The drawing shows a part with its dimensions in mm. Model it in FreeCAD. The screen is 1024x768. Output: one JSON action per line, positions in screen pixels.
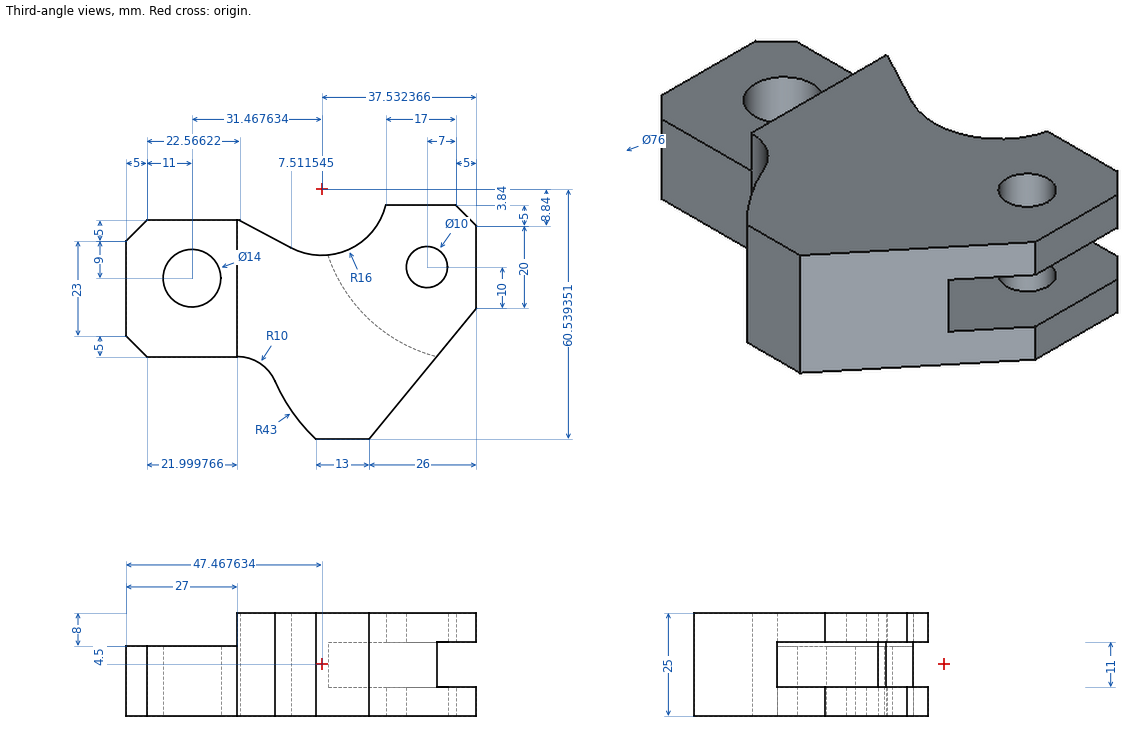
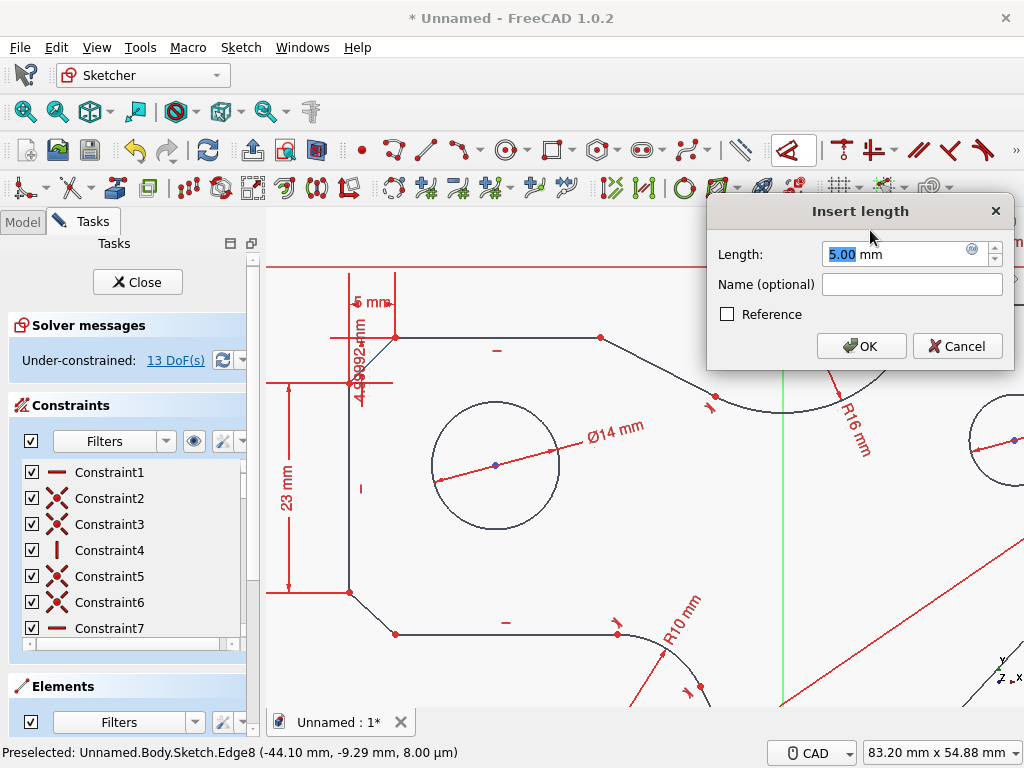
{"action": "type", "text": "5"}
{"action": "key", "text": "Return"}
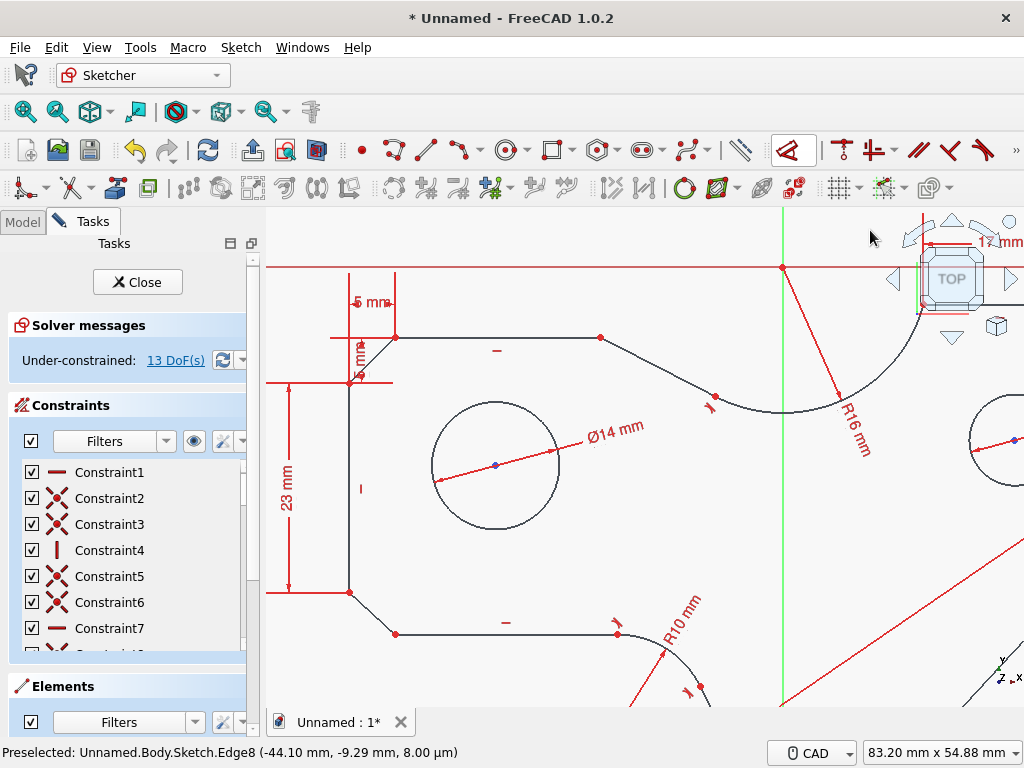
{"action": "left_click", "coordinate": [363, 605]}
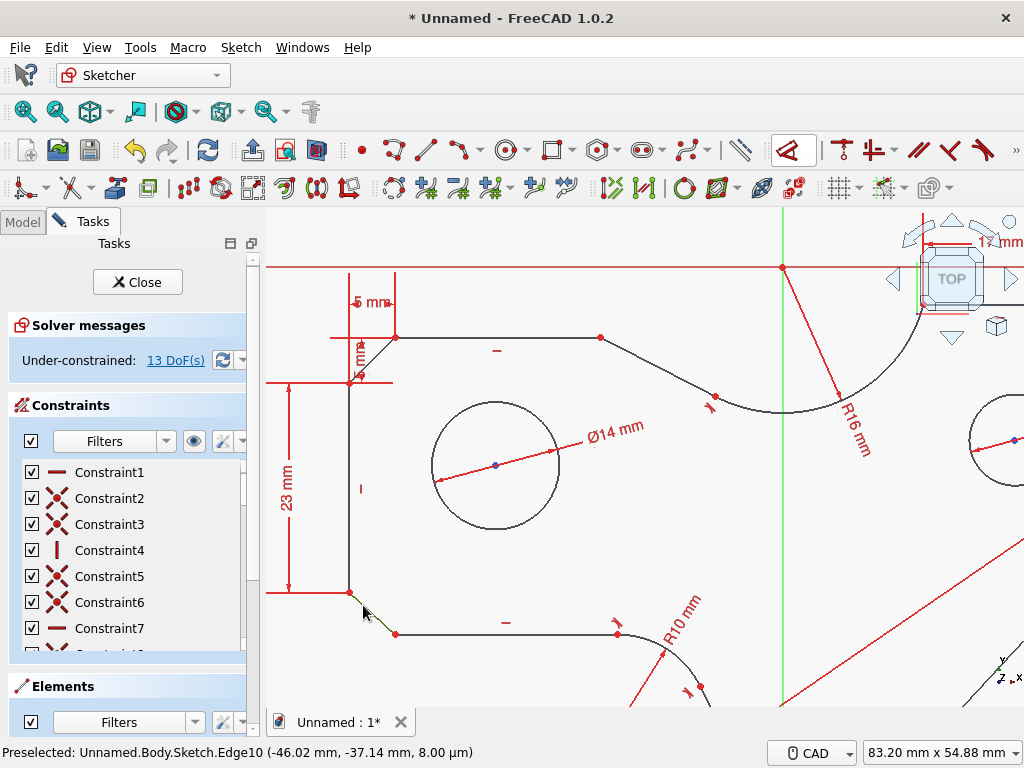
{"action": "key", "text": "l"}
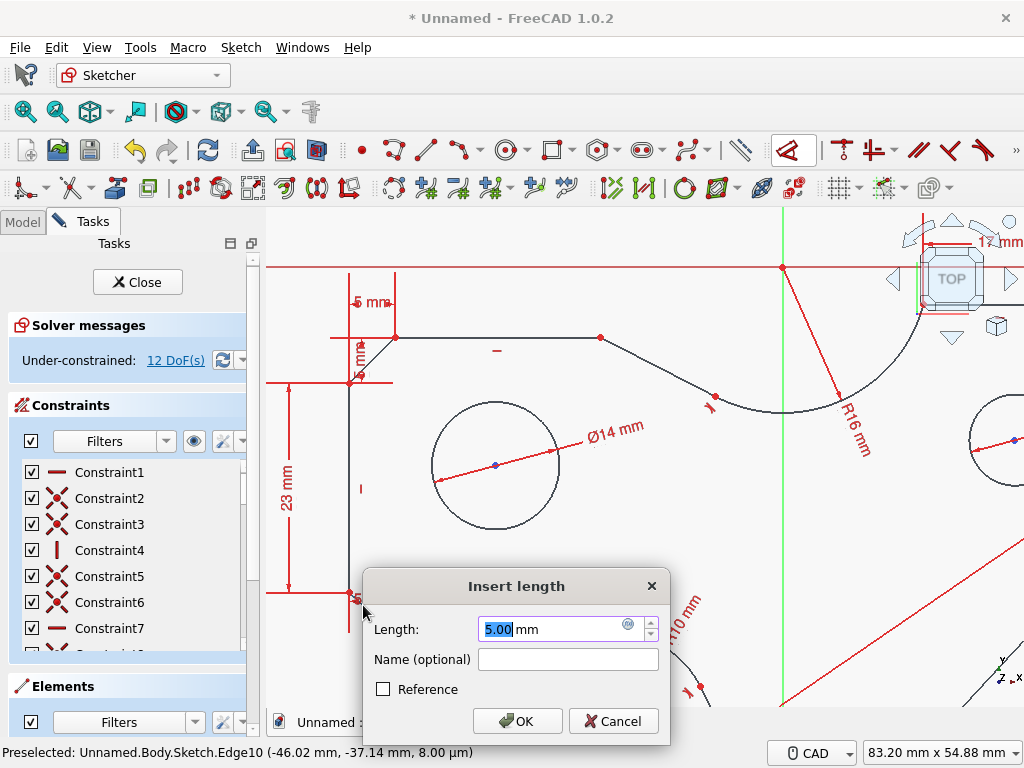
{"action": "type", "text": "5"}
{"action": "key", "text": "Return"}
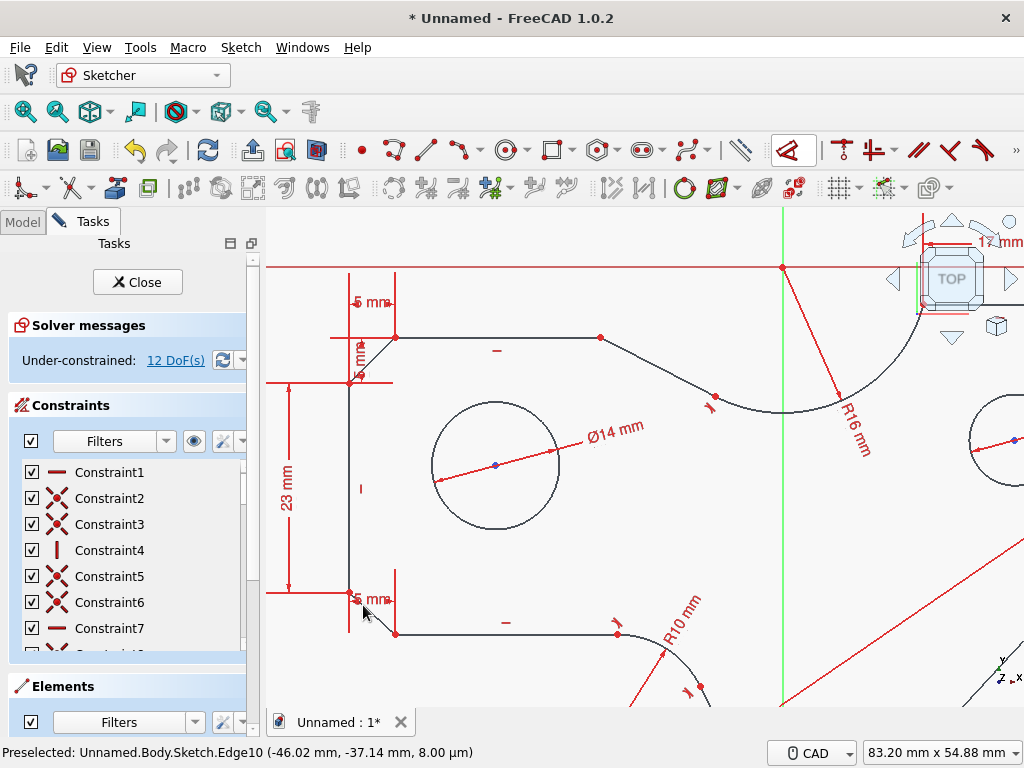
{"action": "left_click", "coordinate": [381, 622]}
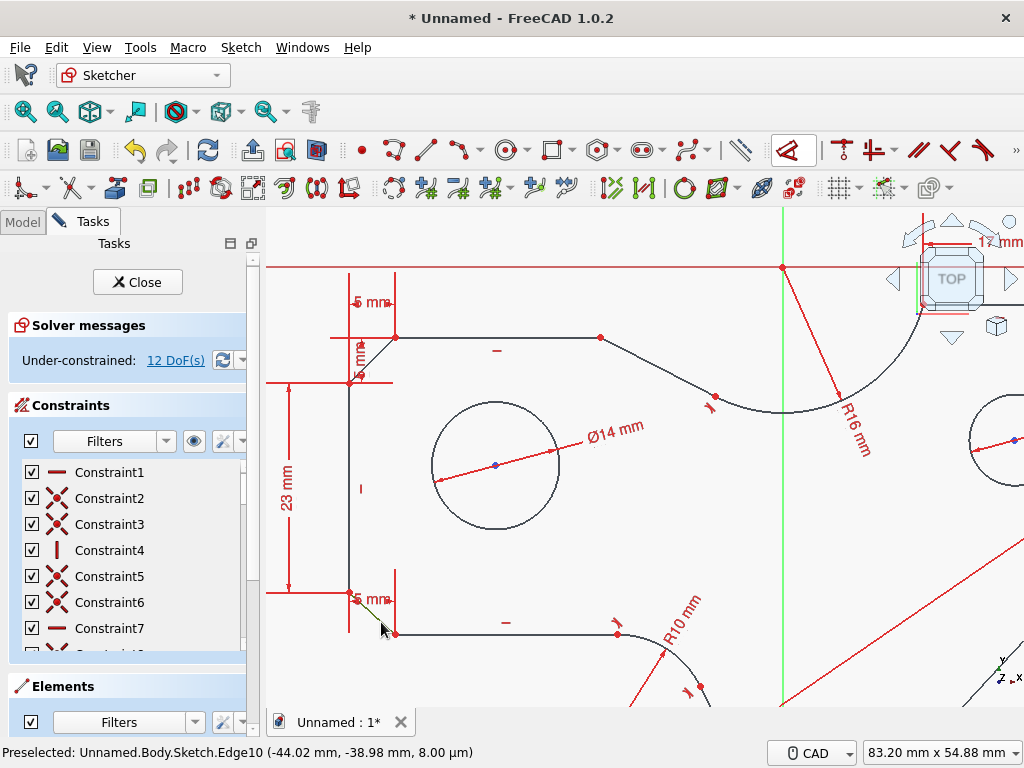
{"action": "left_click", "coordinate": [810, 150]}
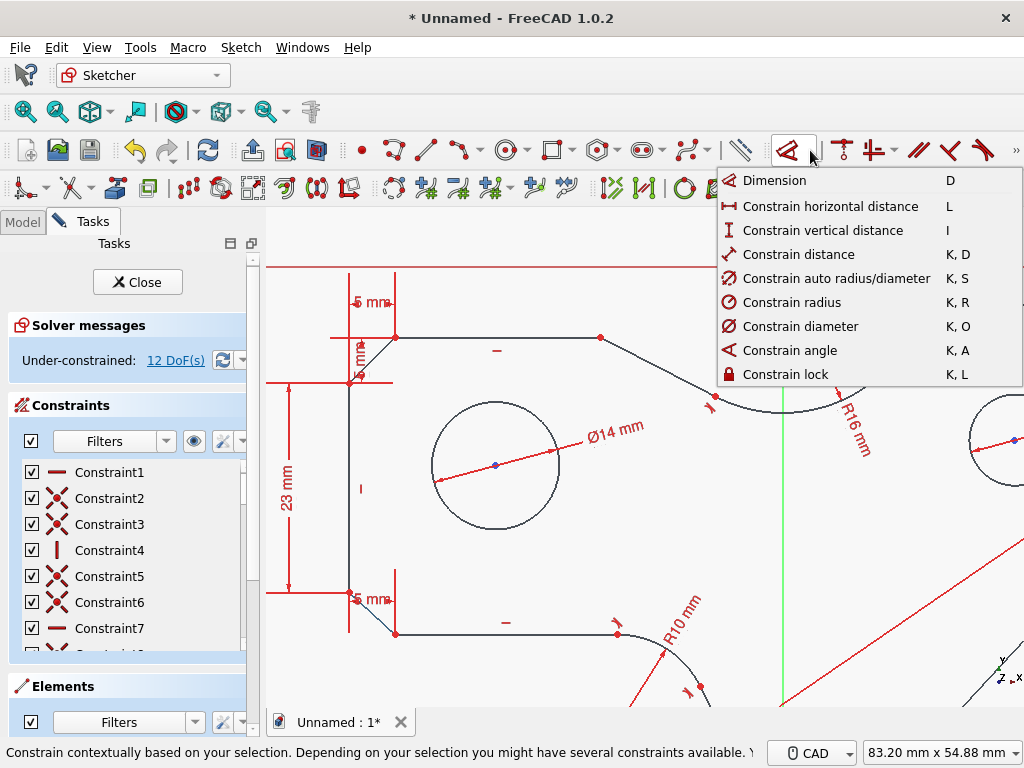
{"action": "left_click", "coordinate": [870, 230]}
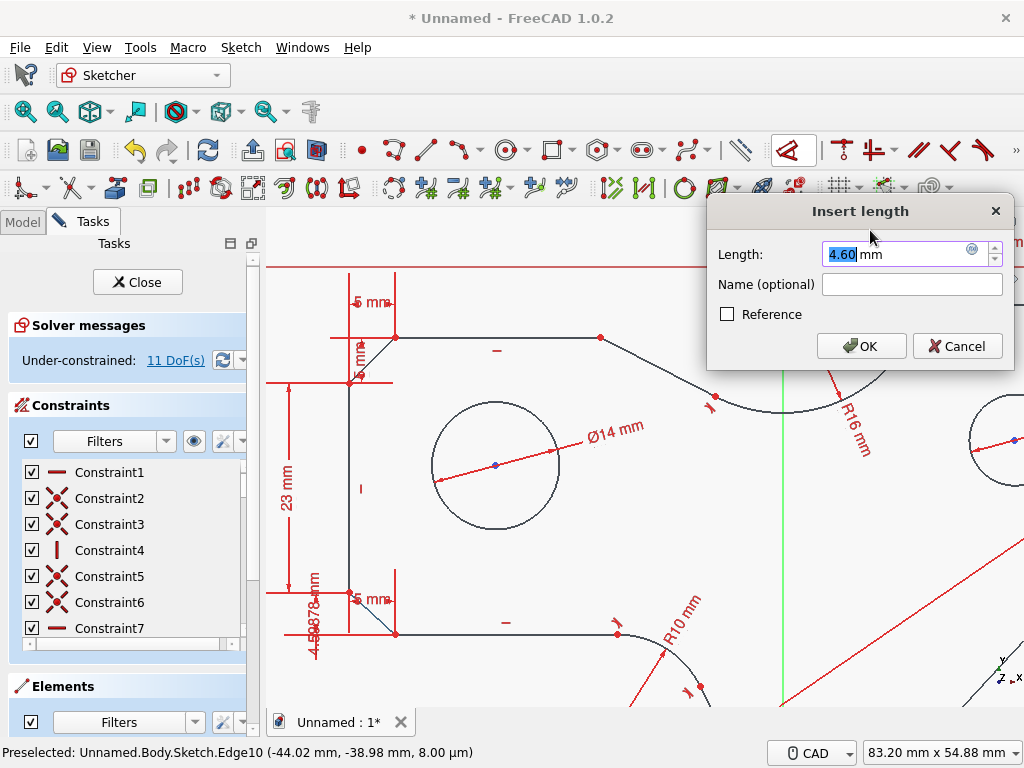
{"action": "type", "text": "5"}
{"action": "key", "text": "Return"}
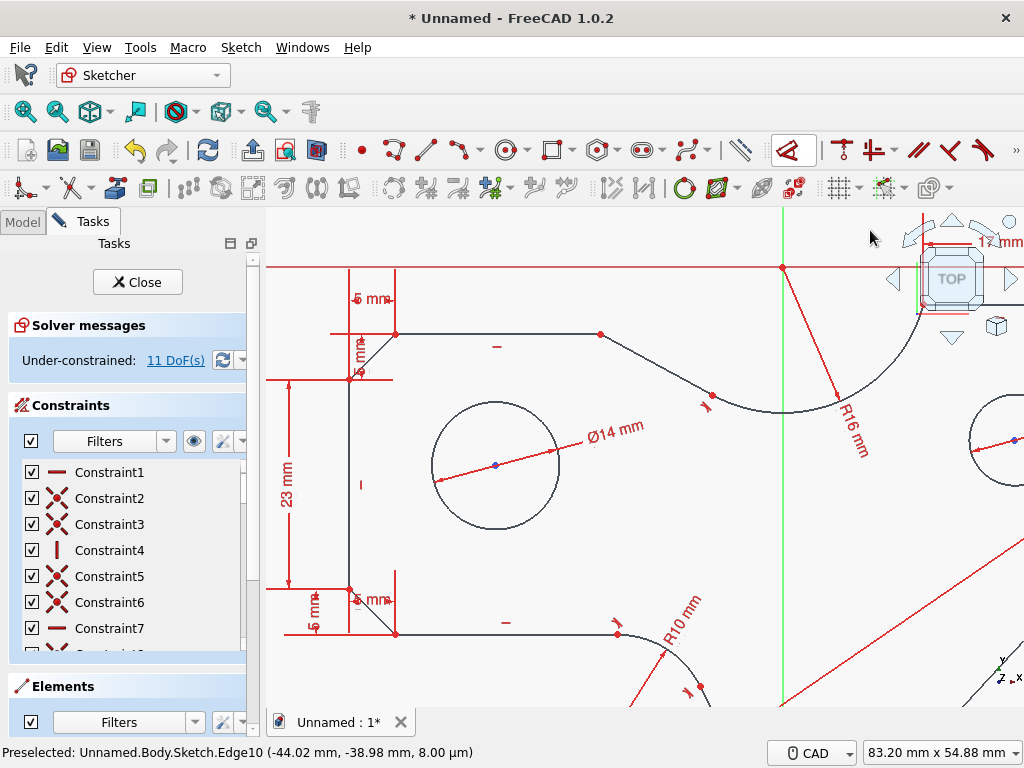
{"action": "left_click", "coordinate": [349, 380]}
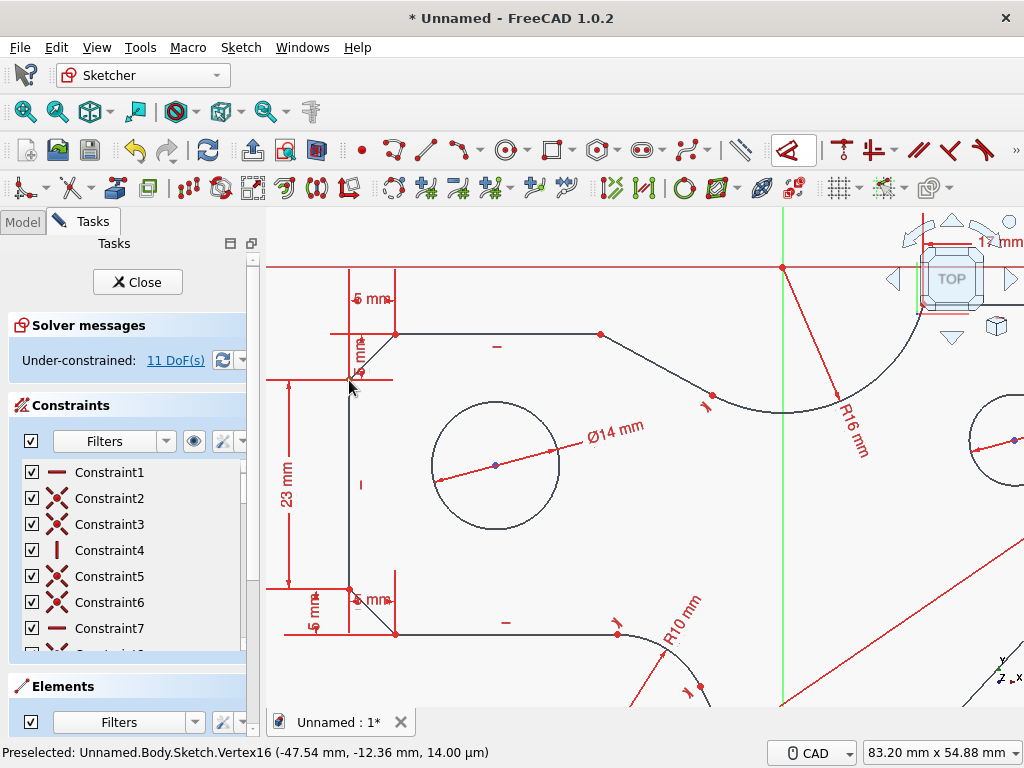
{"action": "left_click", "coordinate": [496, 466]}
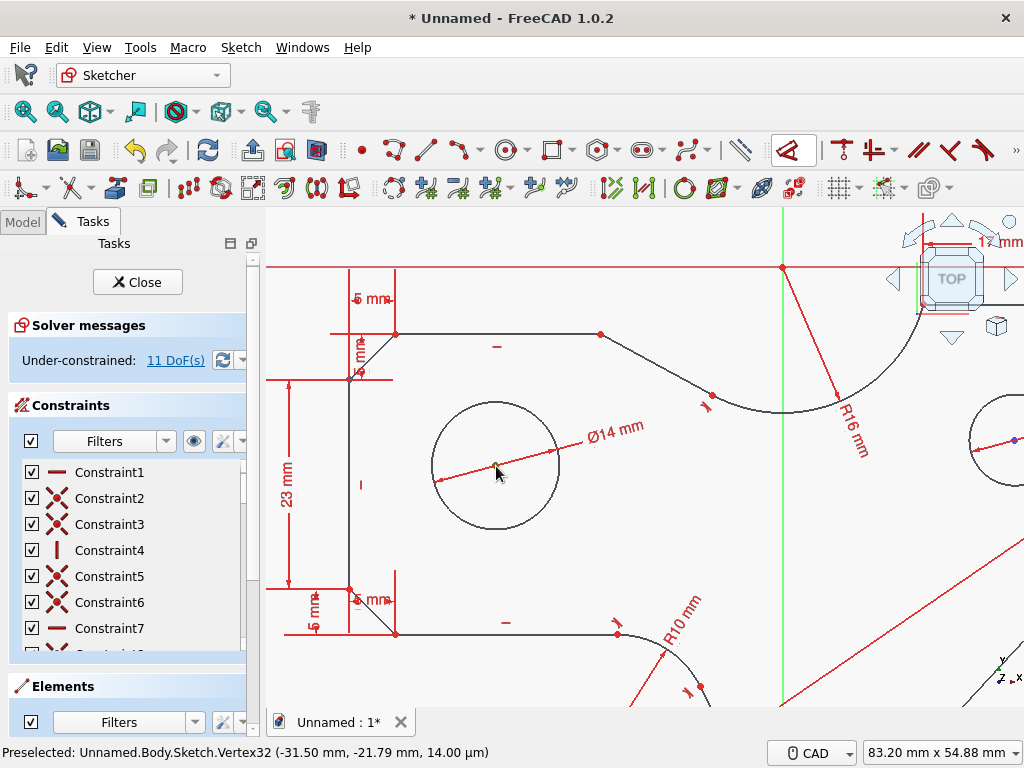
{"action": "key", "text": "i"}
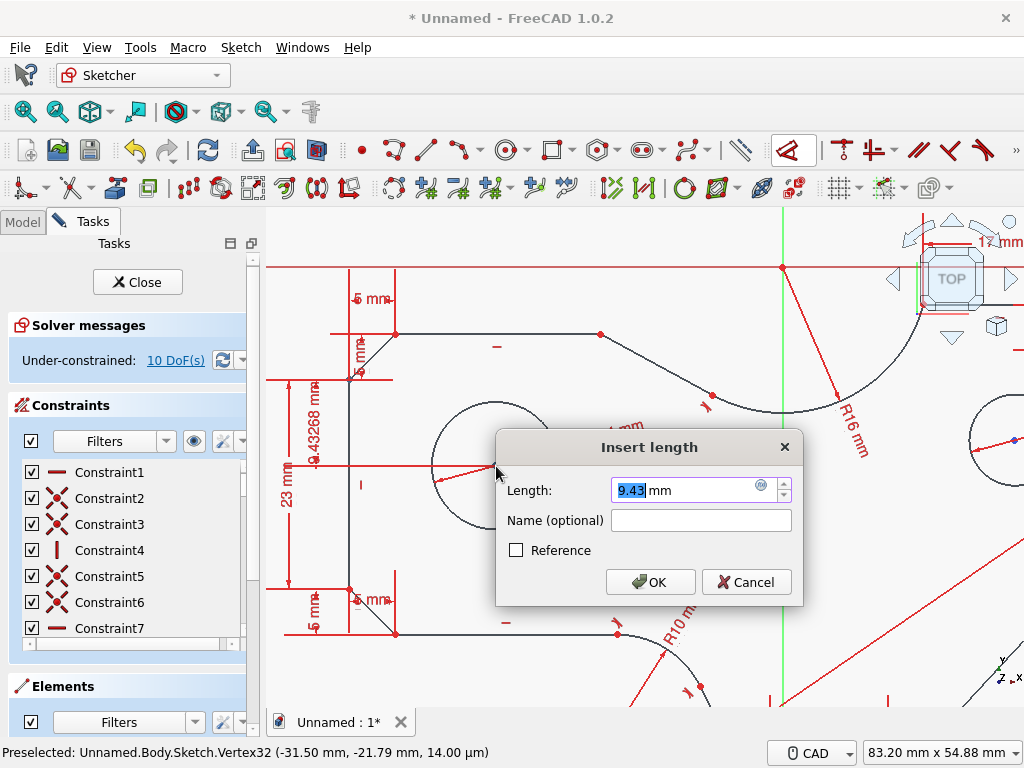
{"action": "type", "text": "9"}
{"action": "key", "text": "Return"}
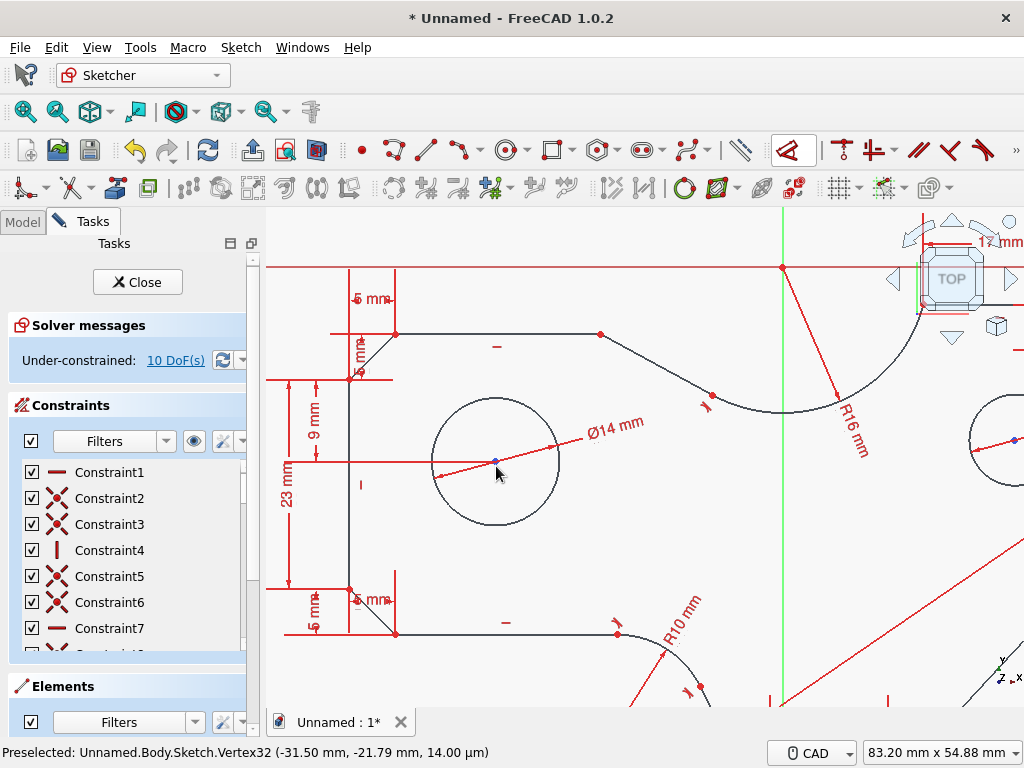
{"action": "scroll", "coordinate": [381, 352], "scroll_direction": "down", "scroll_amount": 3}